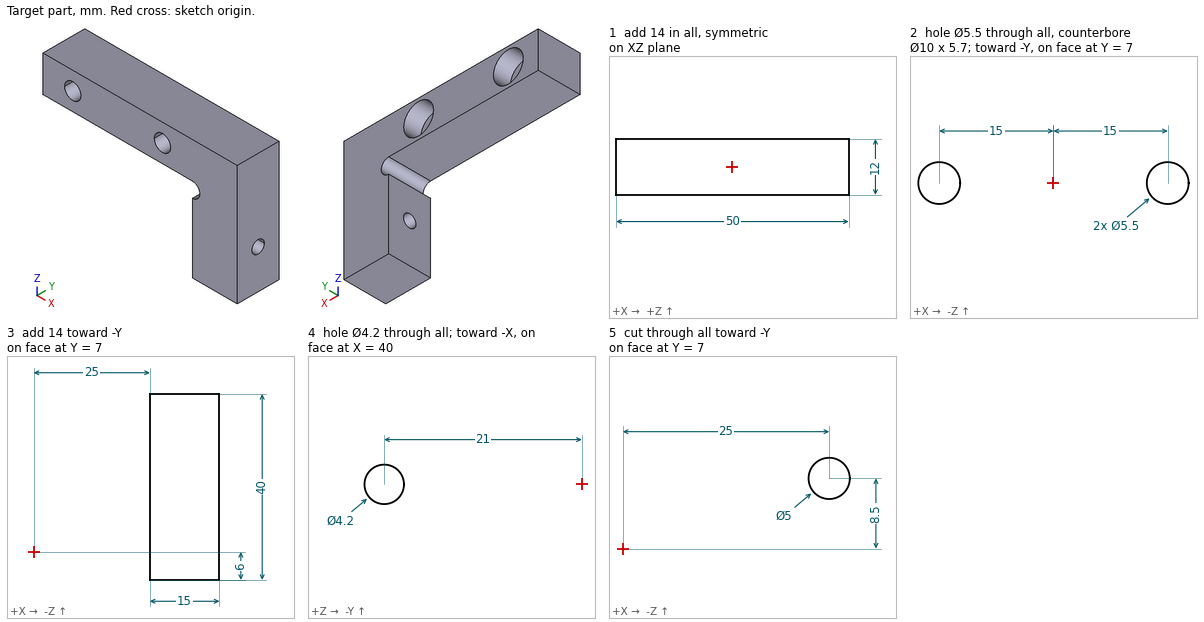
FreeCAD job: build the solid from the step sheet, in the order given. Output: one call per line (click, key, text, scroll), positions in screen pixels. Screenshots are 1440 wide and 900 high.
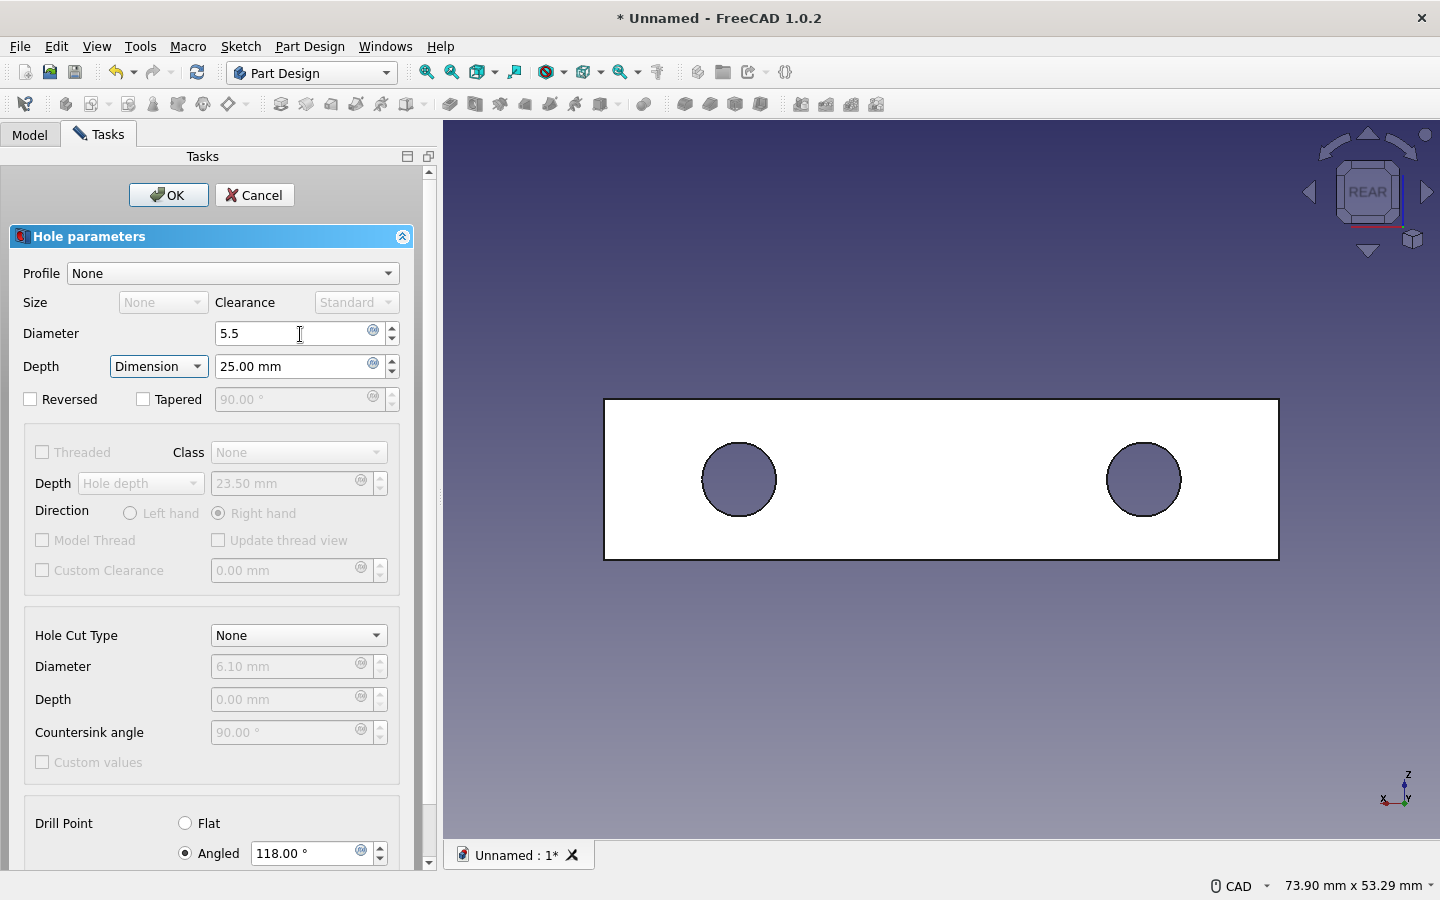
click(160, 366)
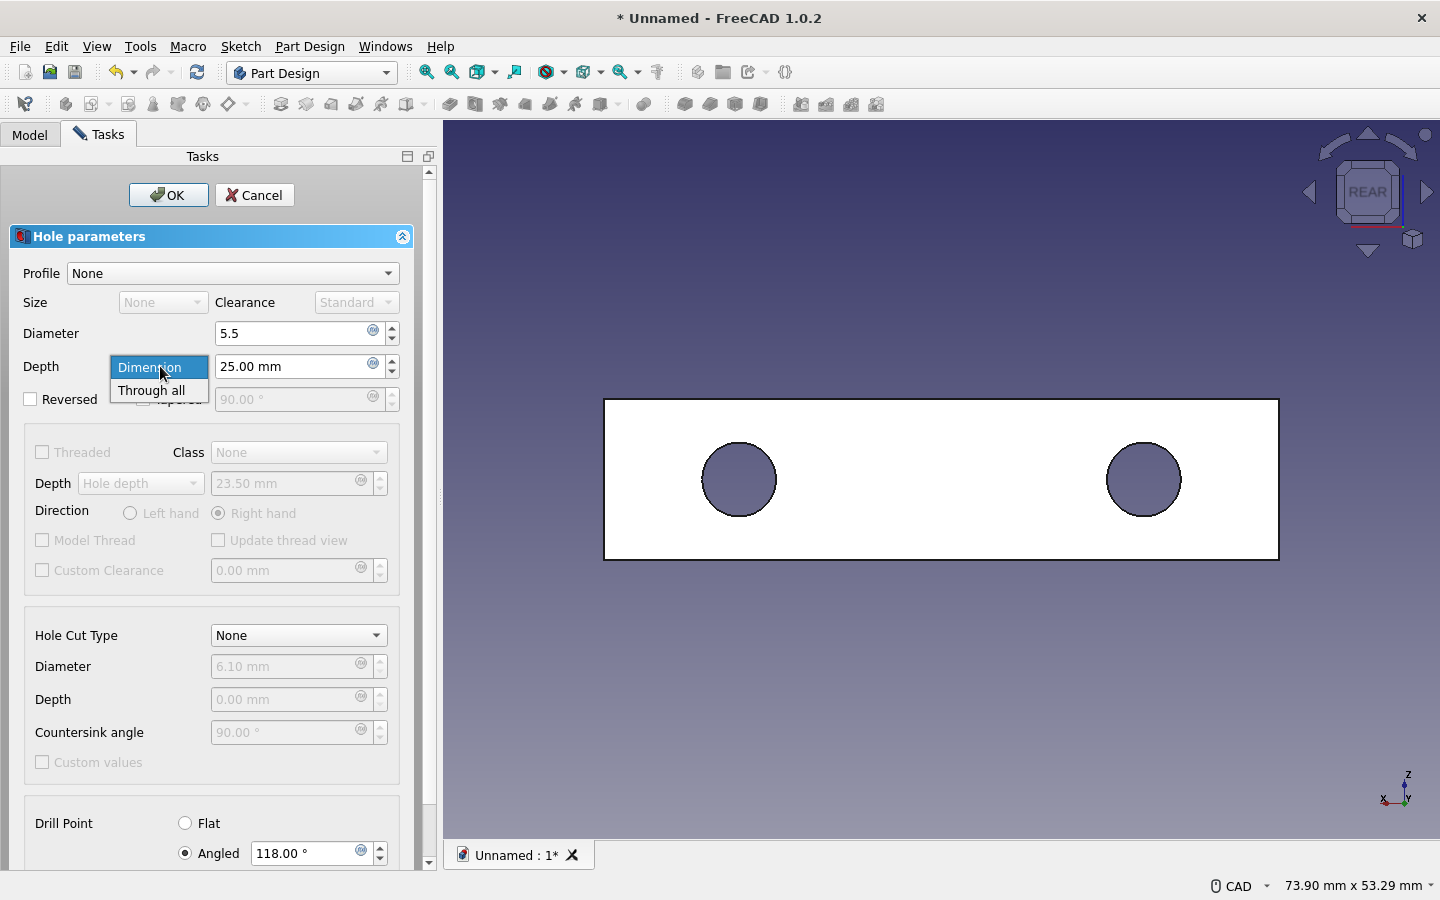
click(158, 390)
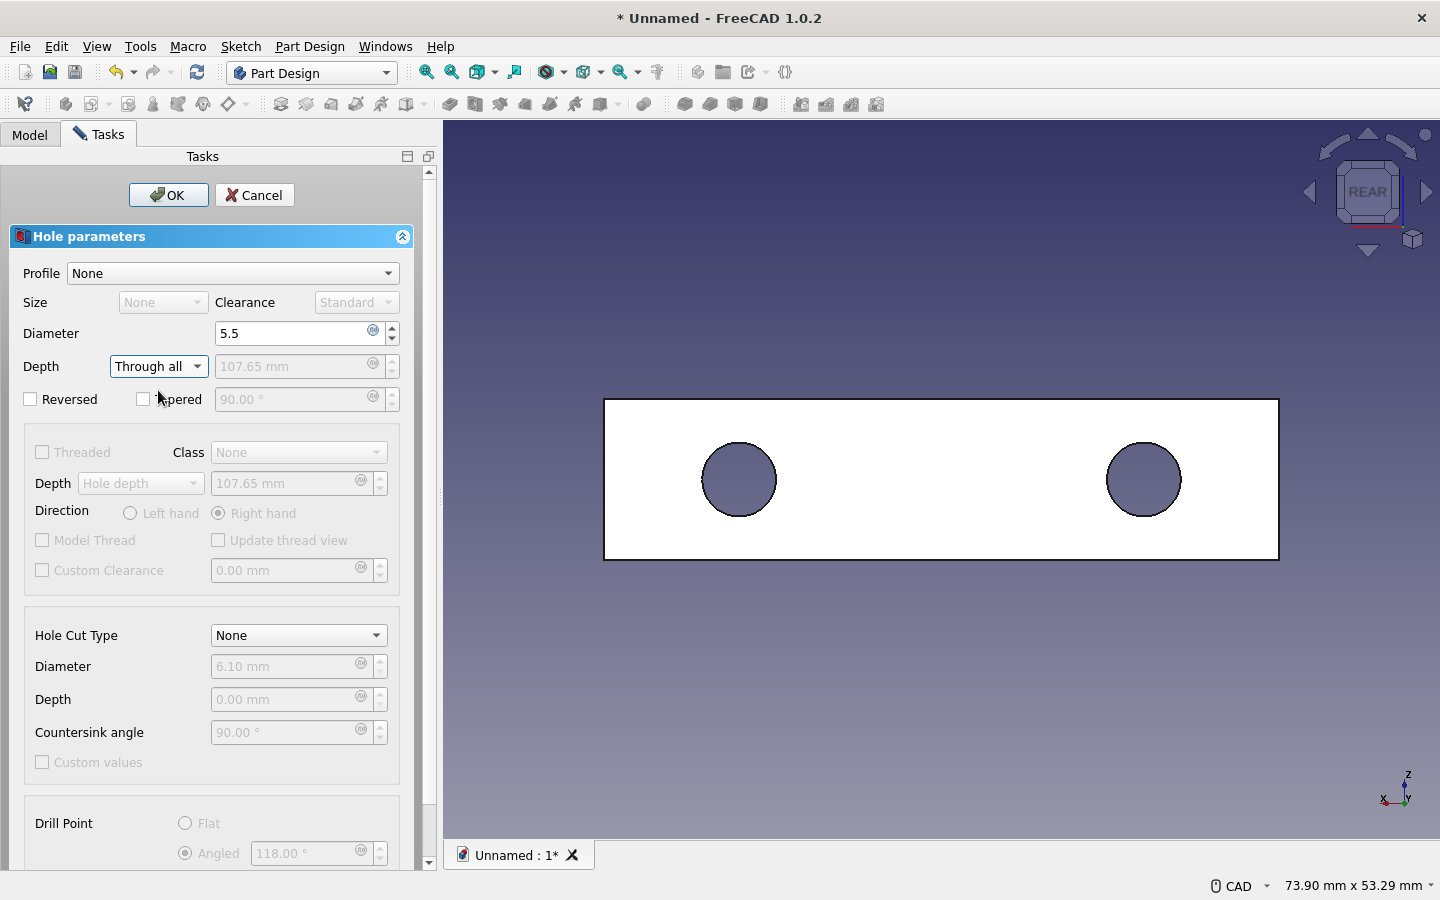
click(300, 636)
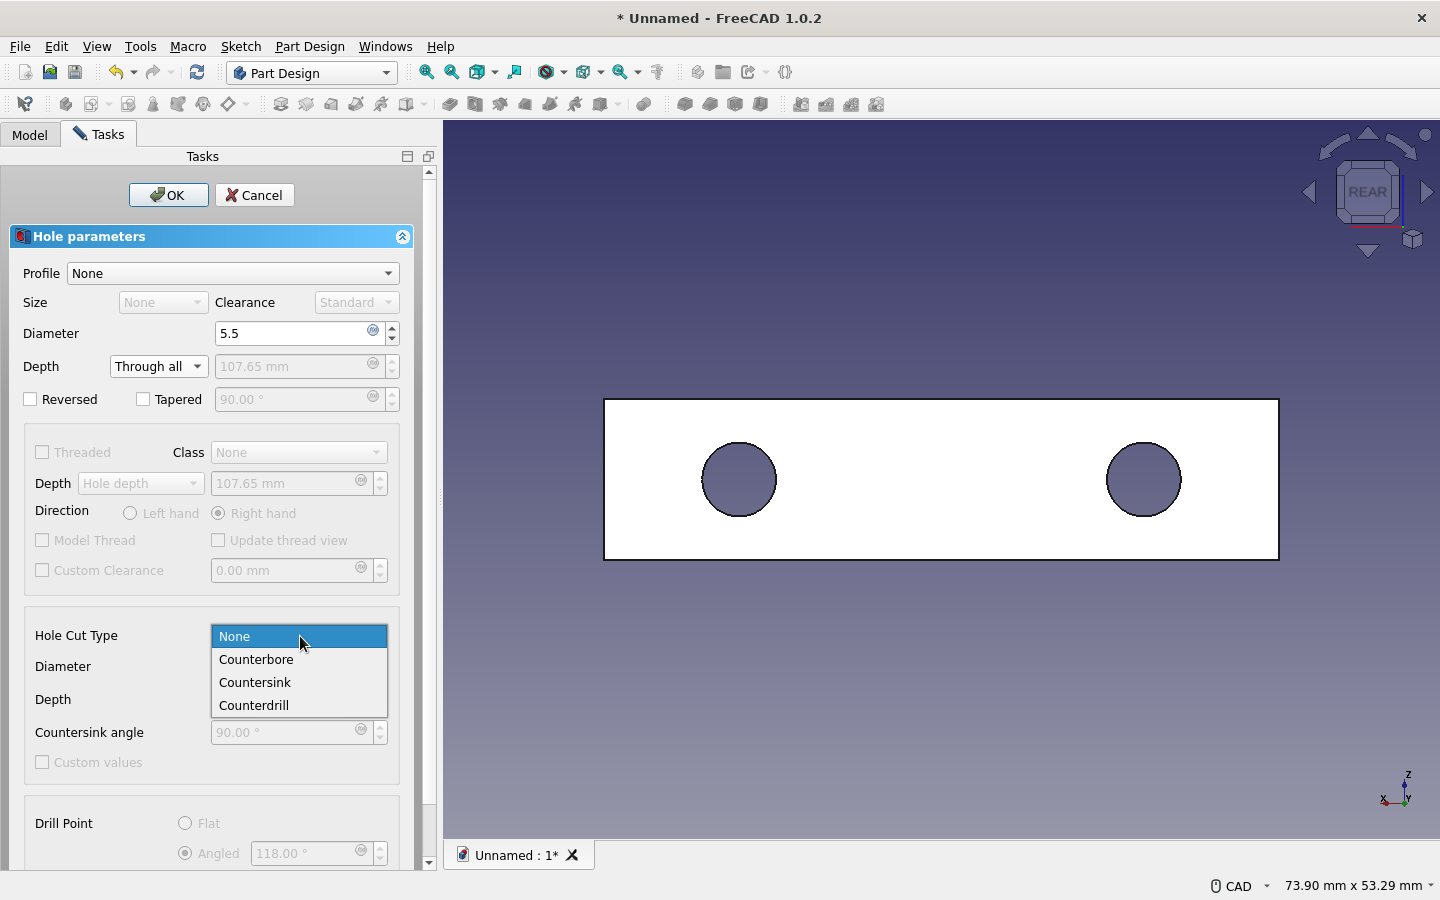
click(298, 660)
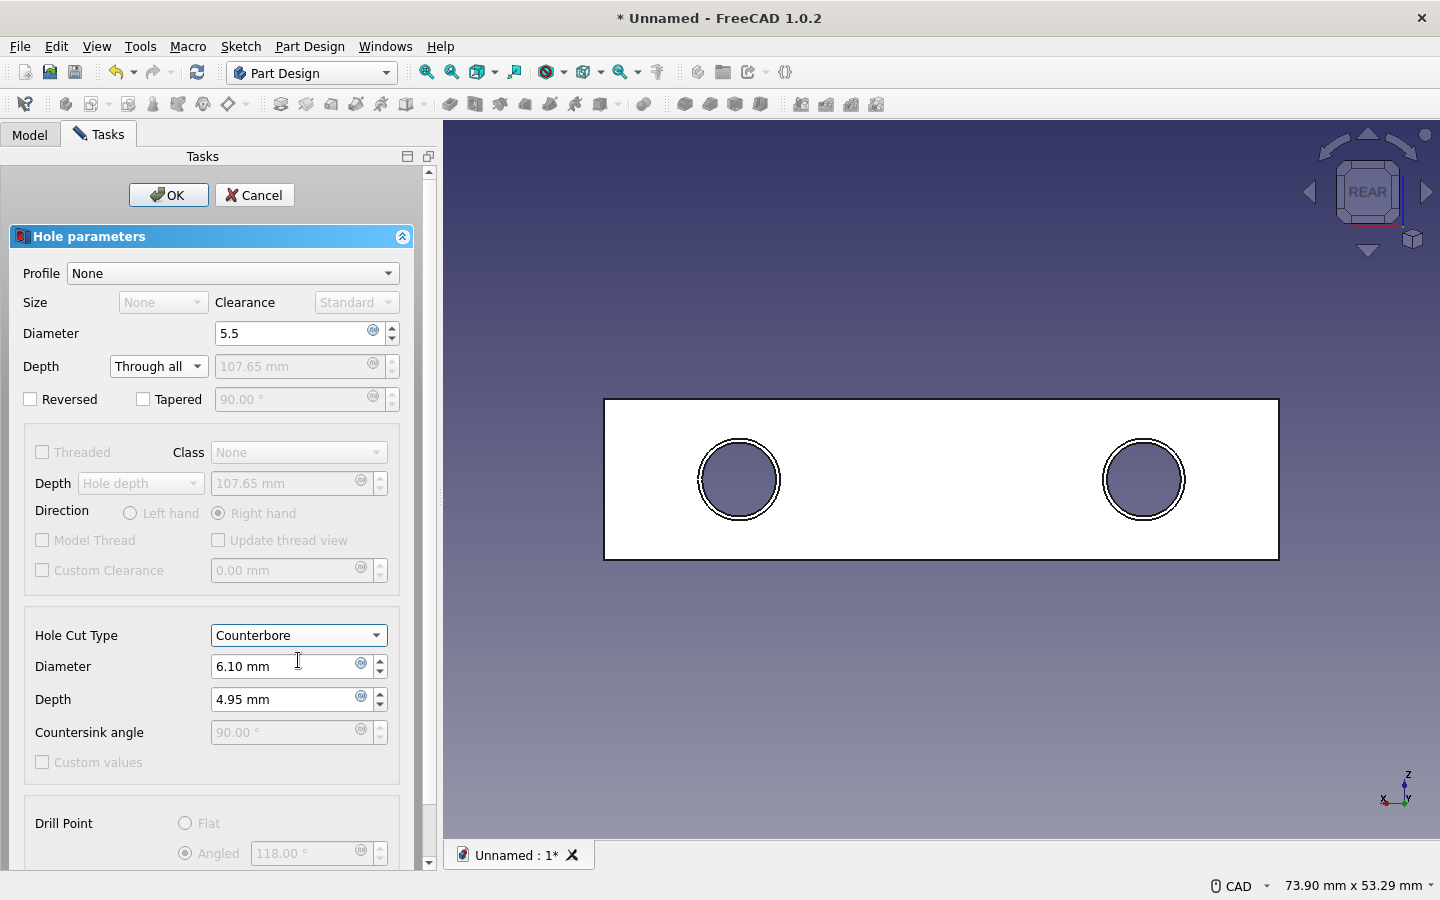
triple_click(292, 666)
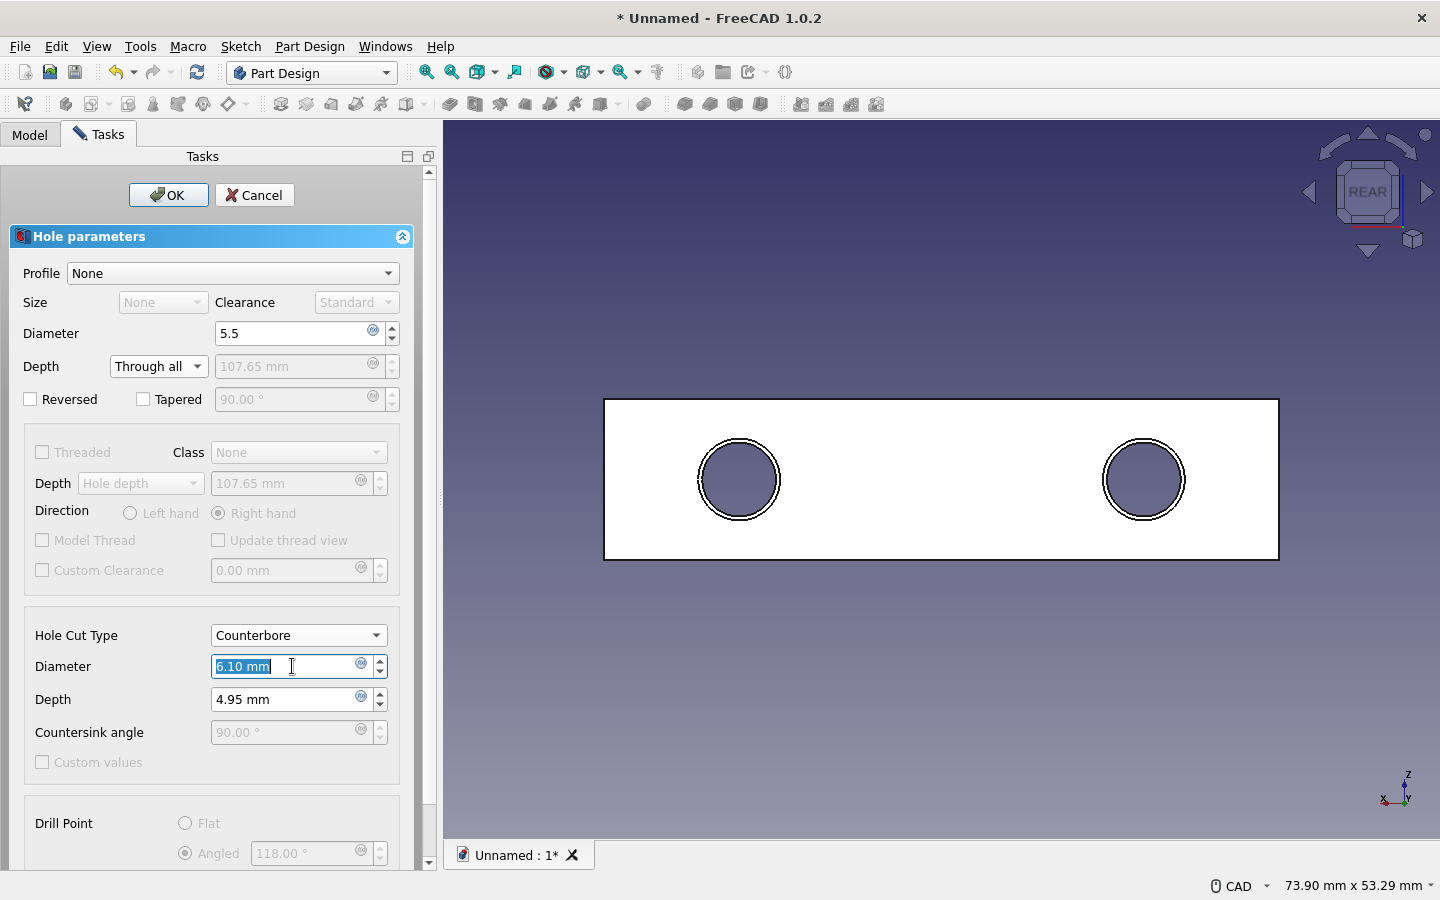
text(10)
key(Tab)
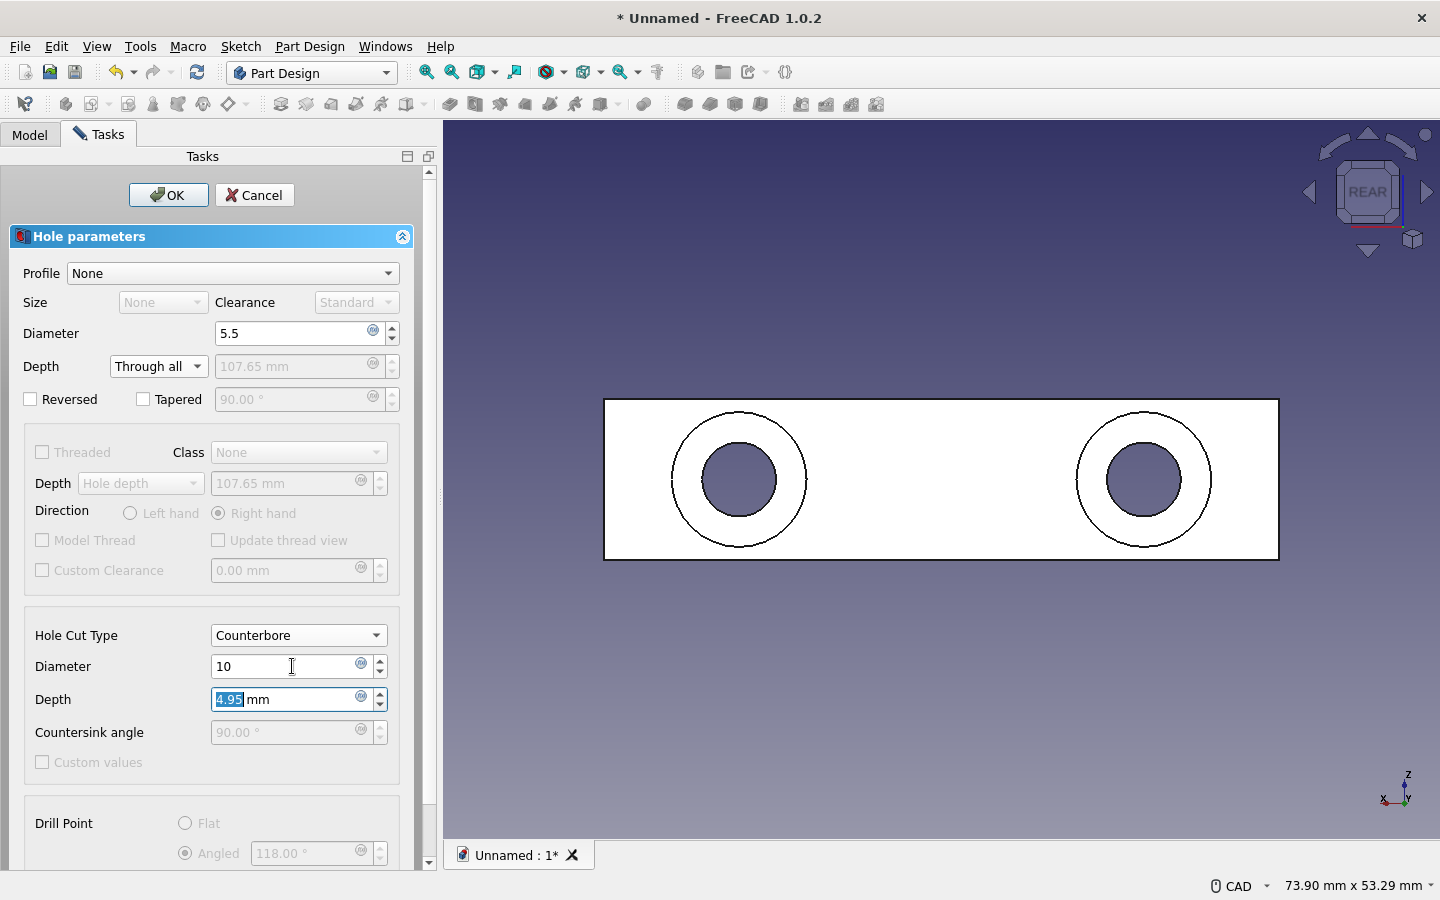
text(5.7)
key(Tab)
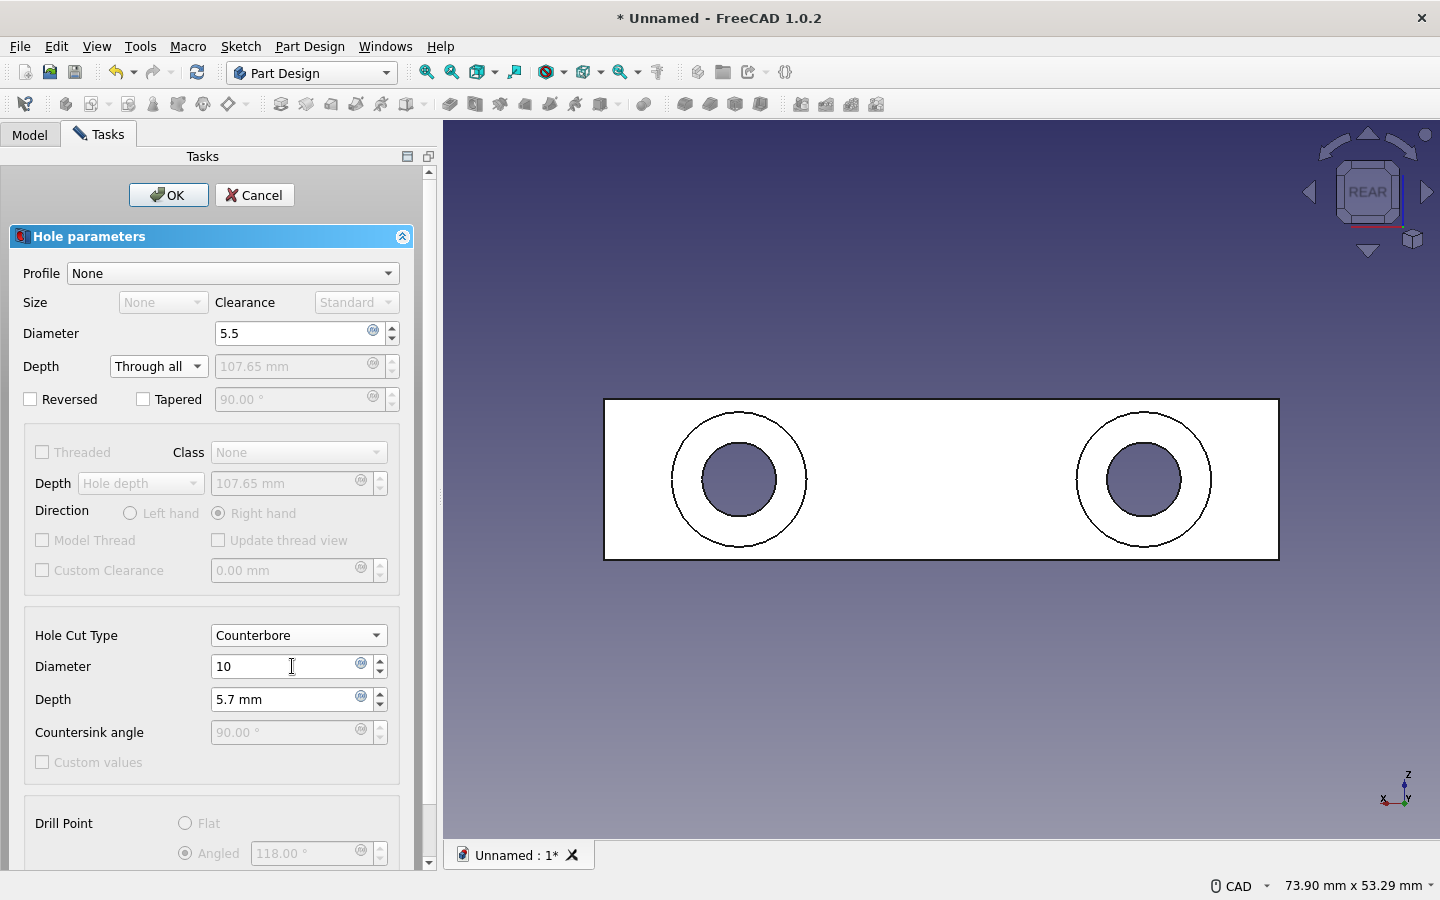
click(169, 195)